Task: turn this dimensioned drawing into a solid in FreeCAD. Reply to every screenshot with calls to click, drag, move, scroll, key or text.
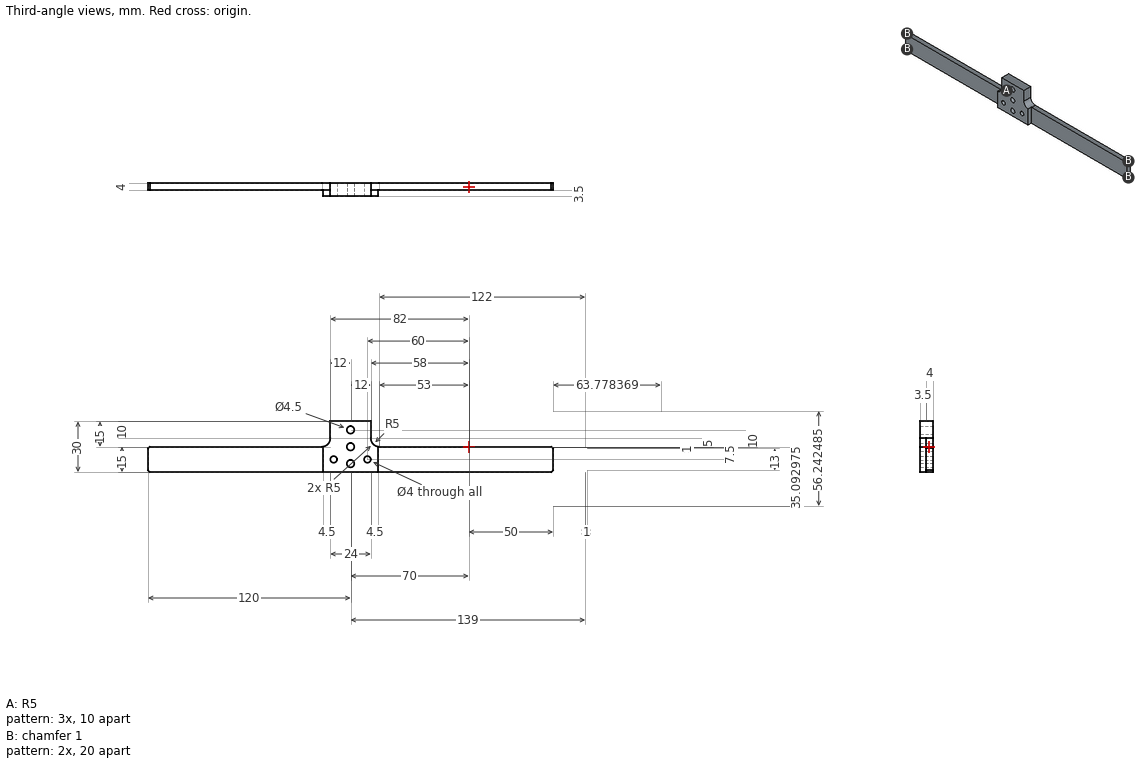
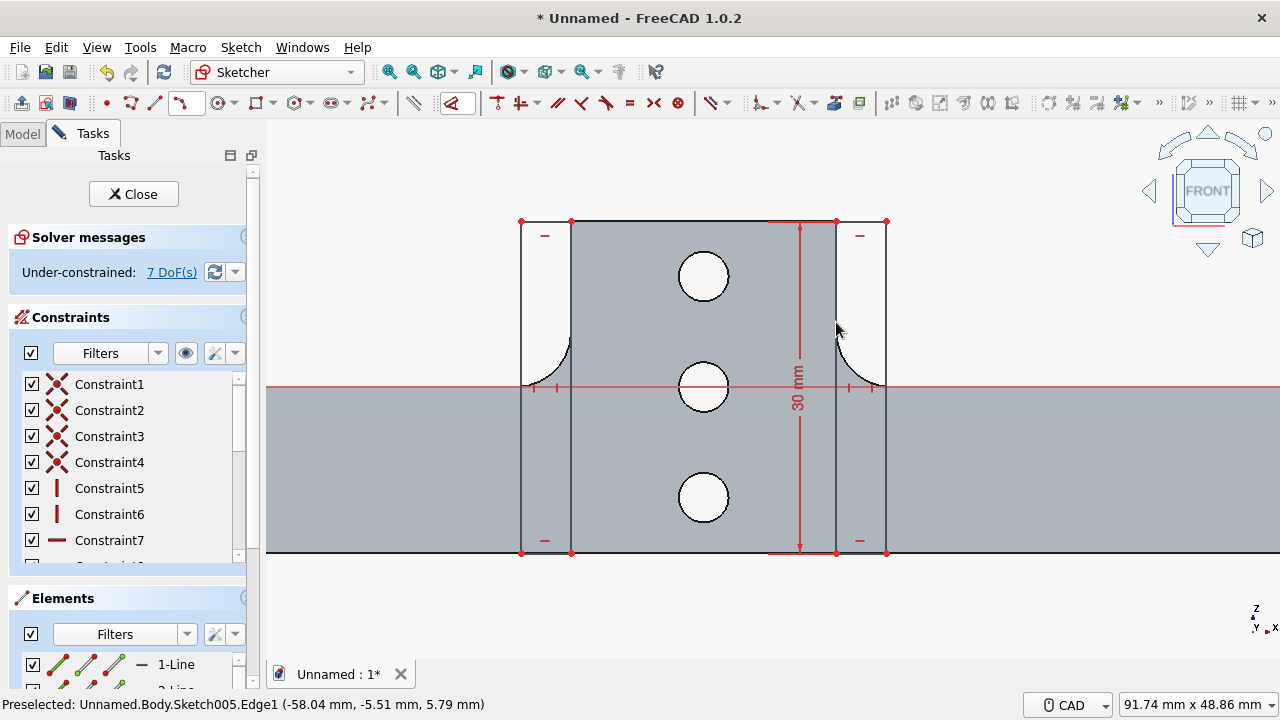
click(521, 322)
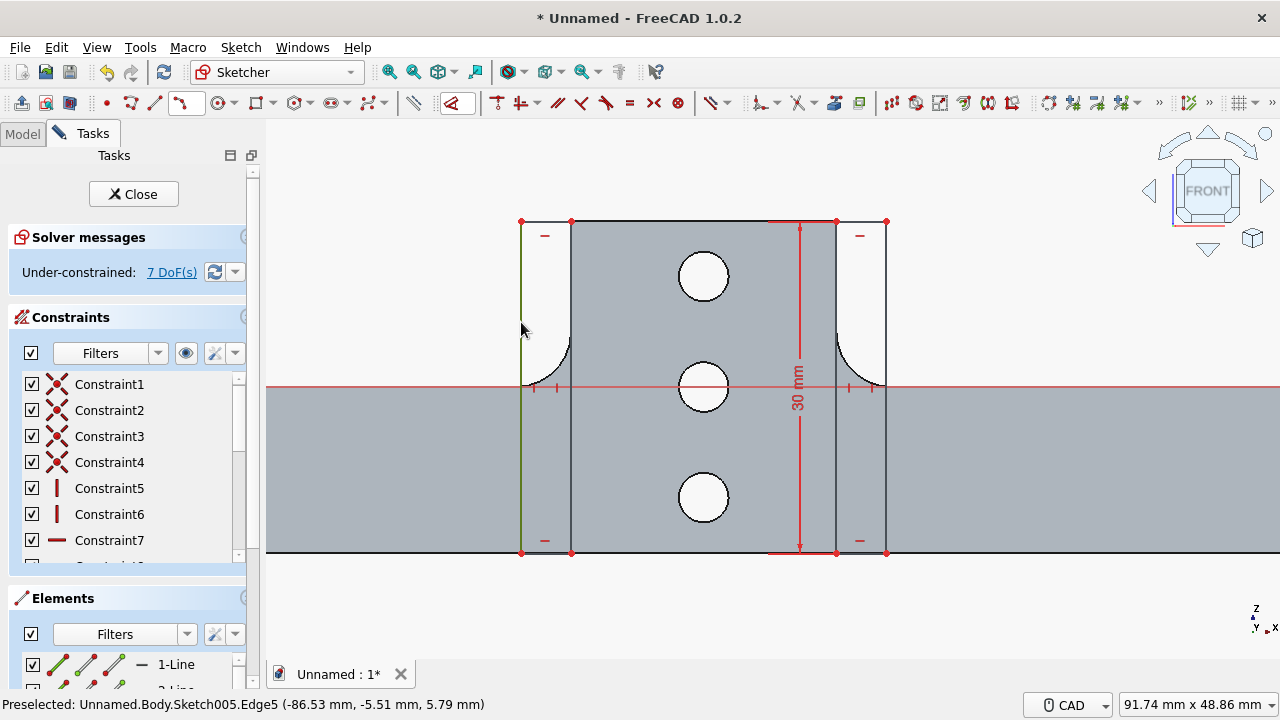
click(470, 104)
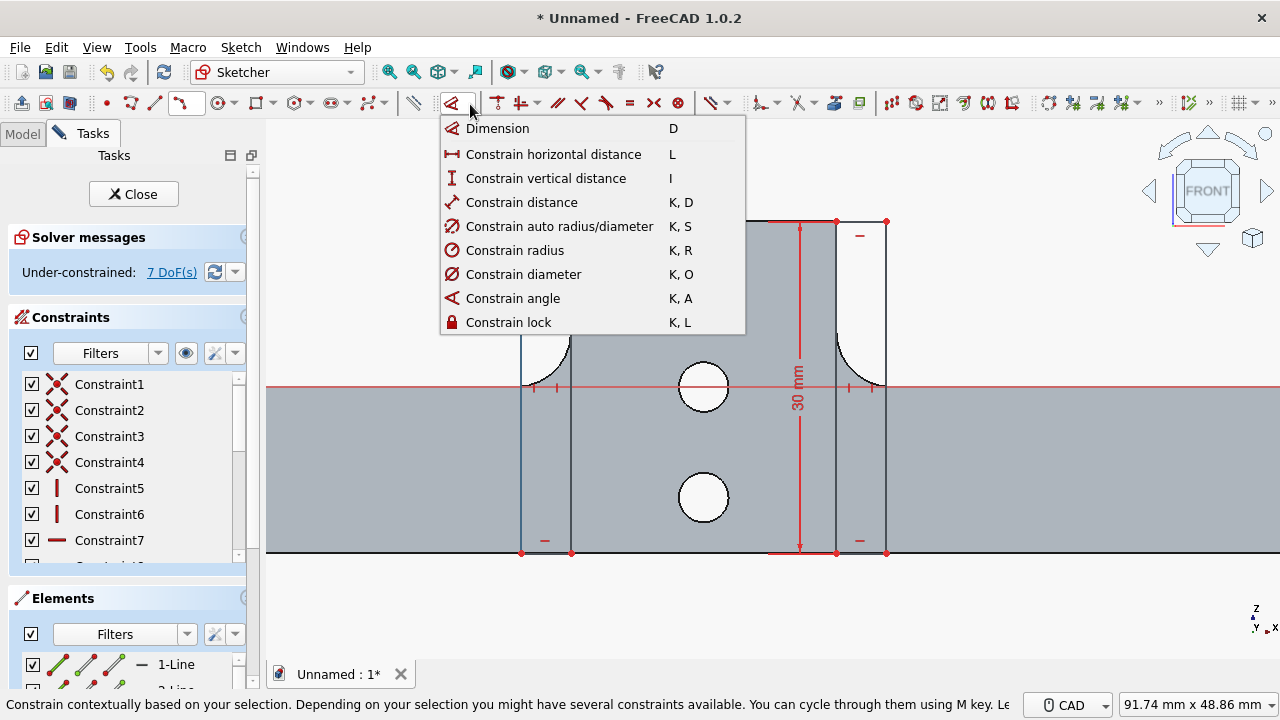
click(593, 178)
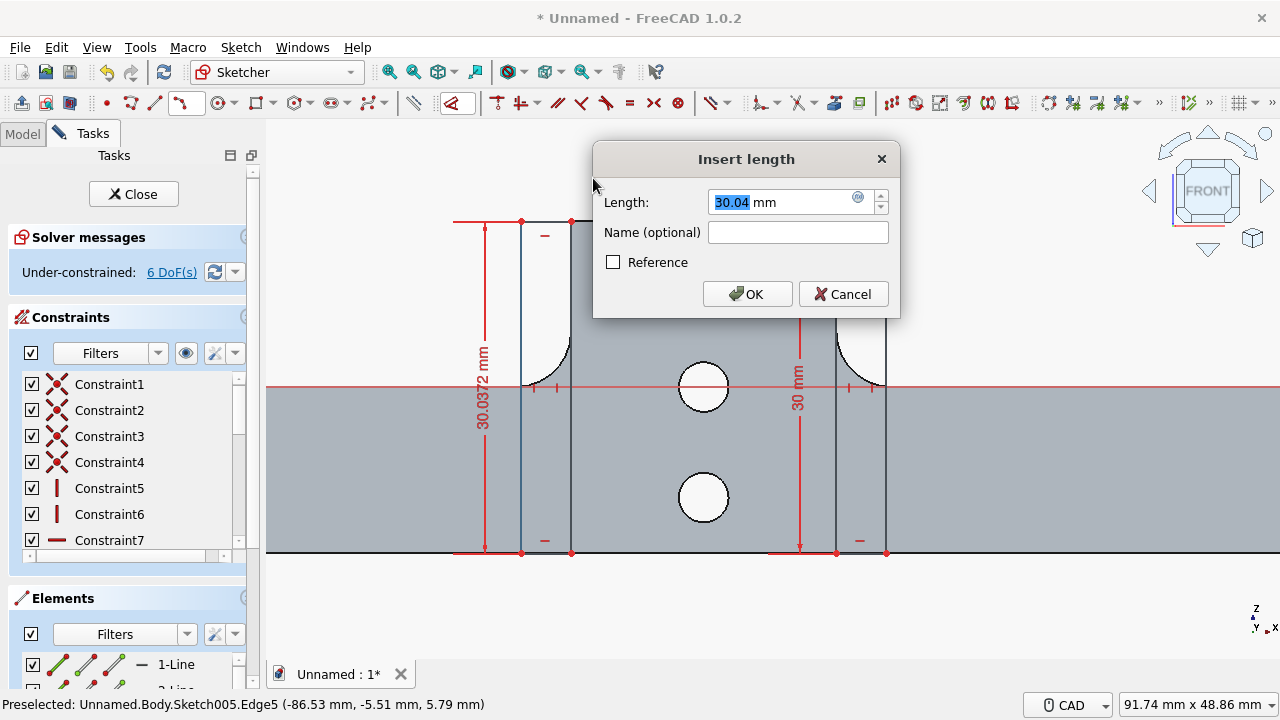
text(30)
key(Return)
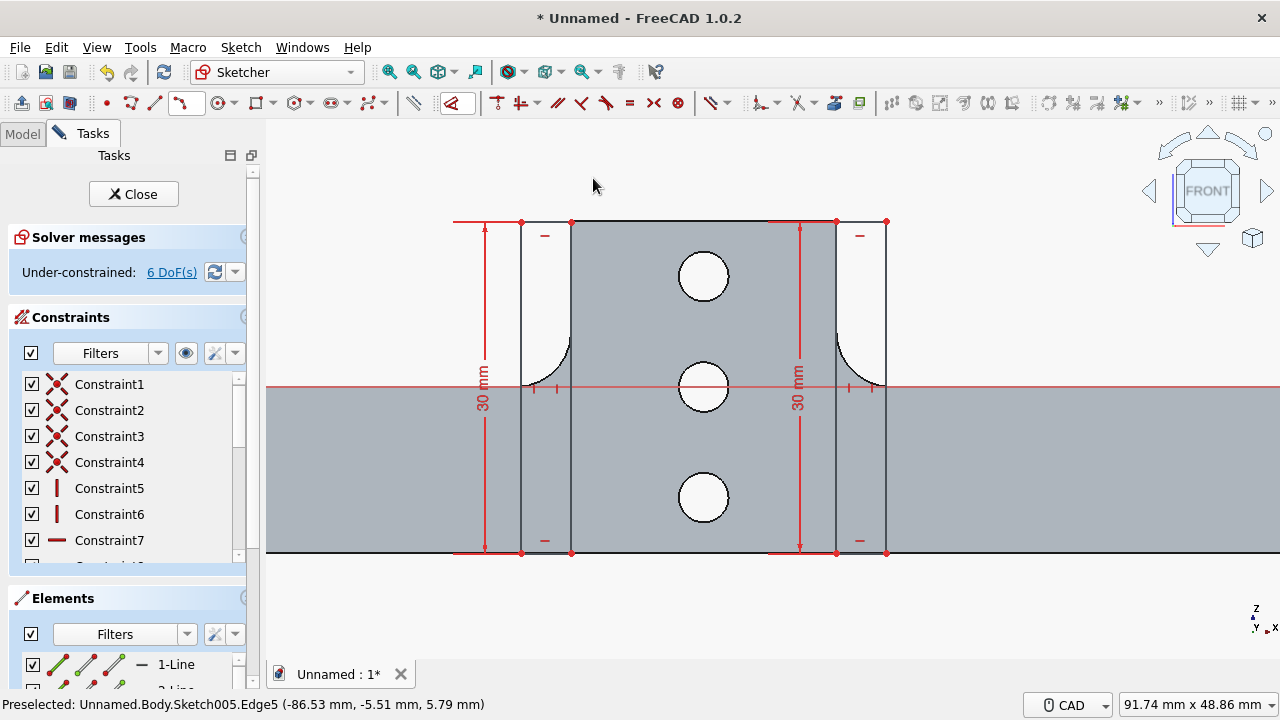
click(851, 554)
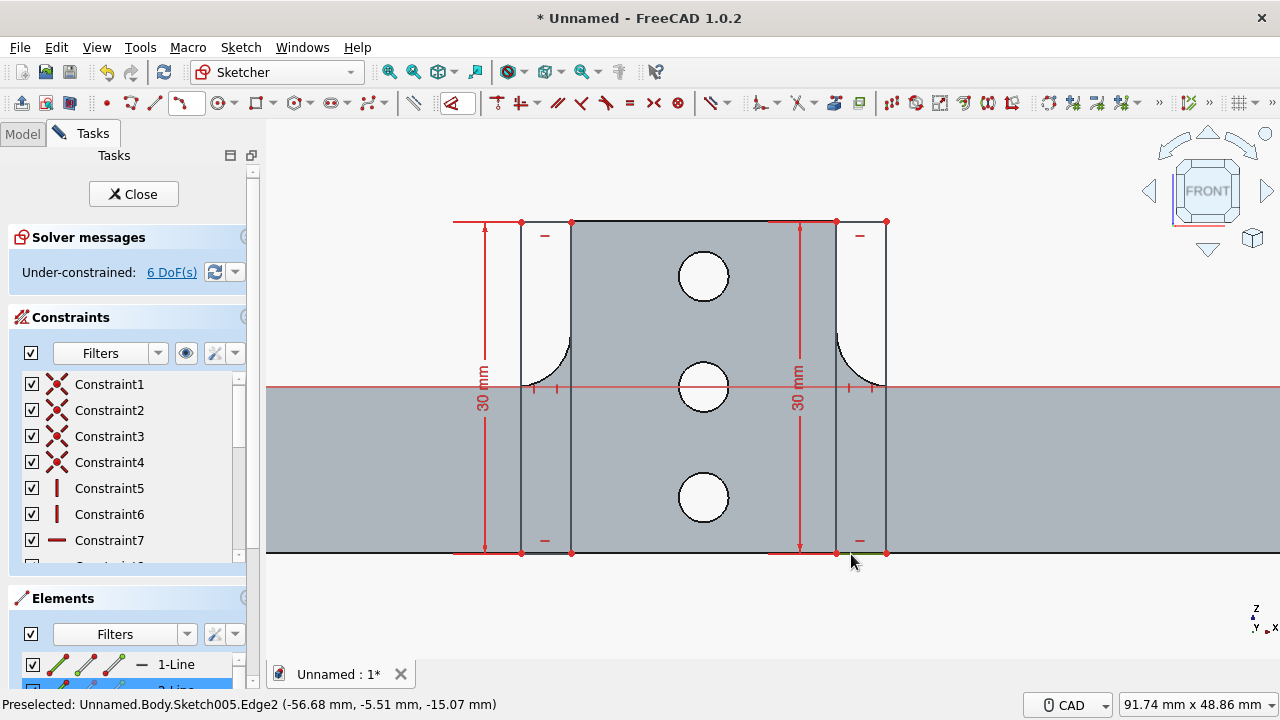
key(l)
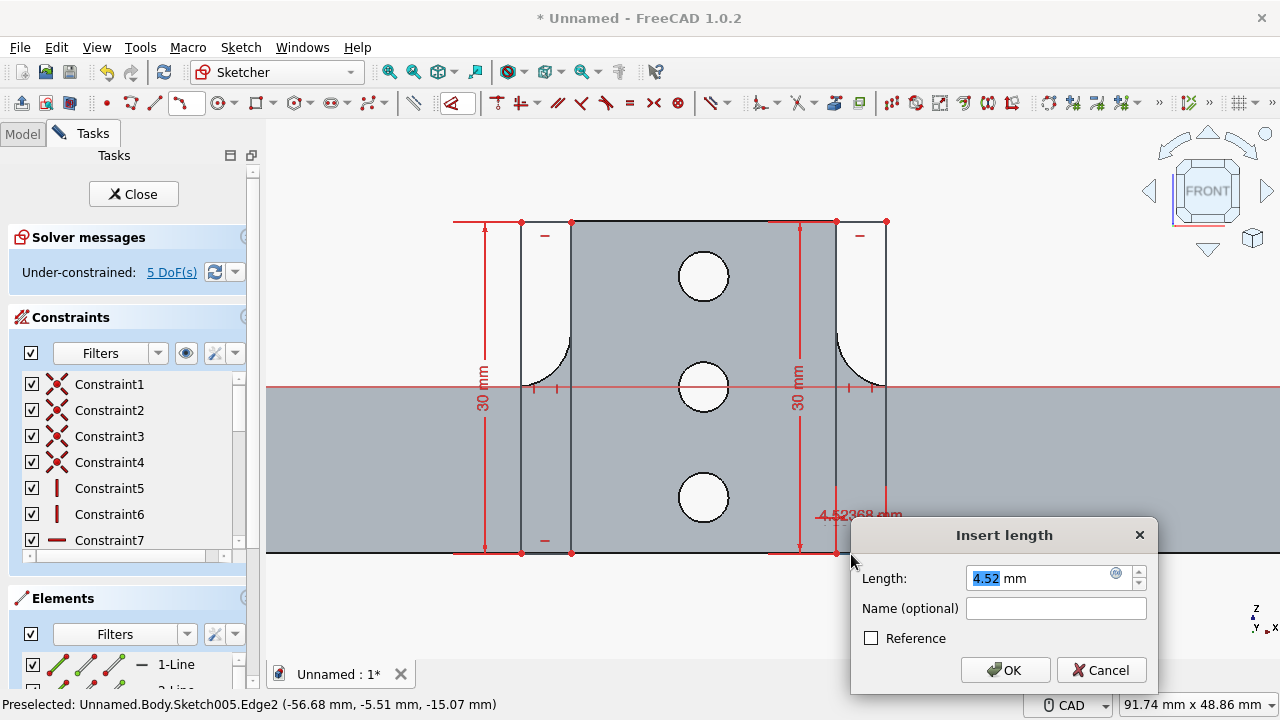
text(4.5)
key(Return)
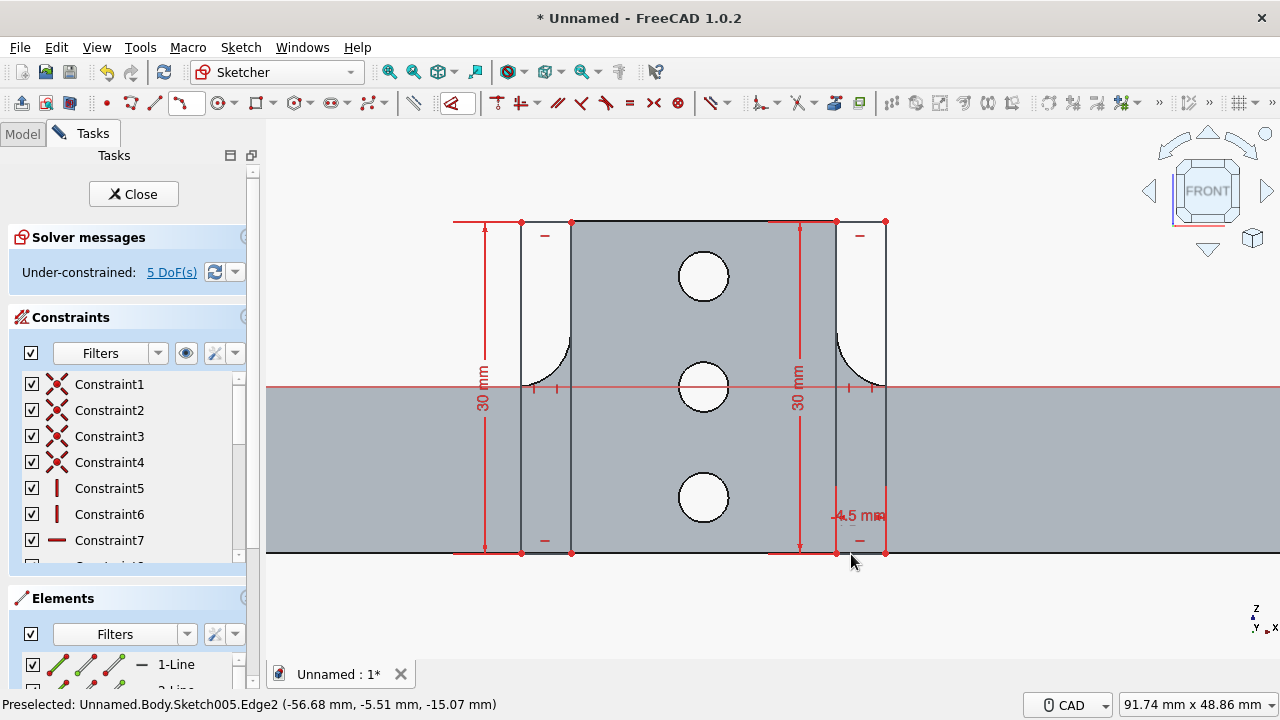
click(536, 554)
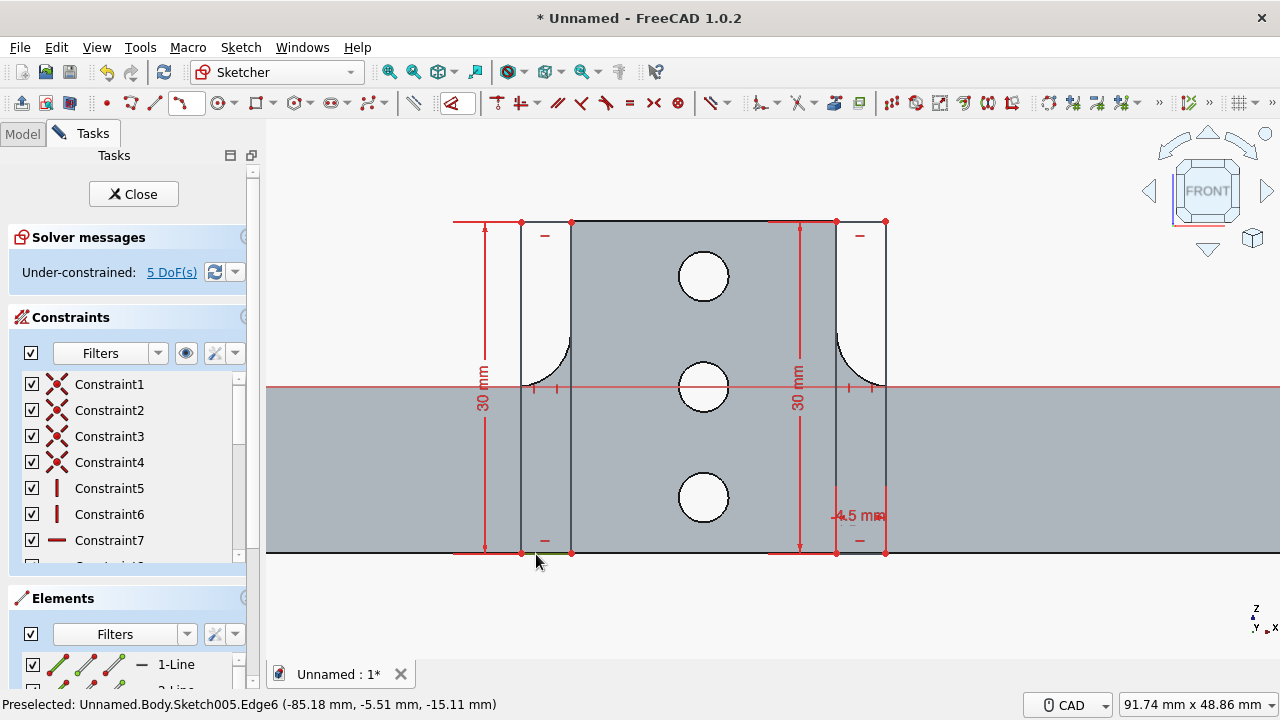
key(l)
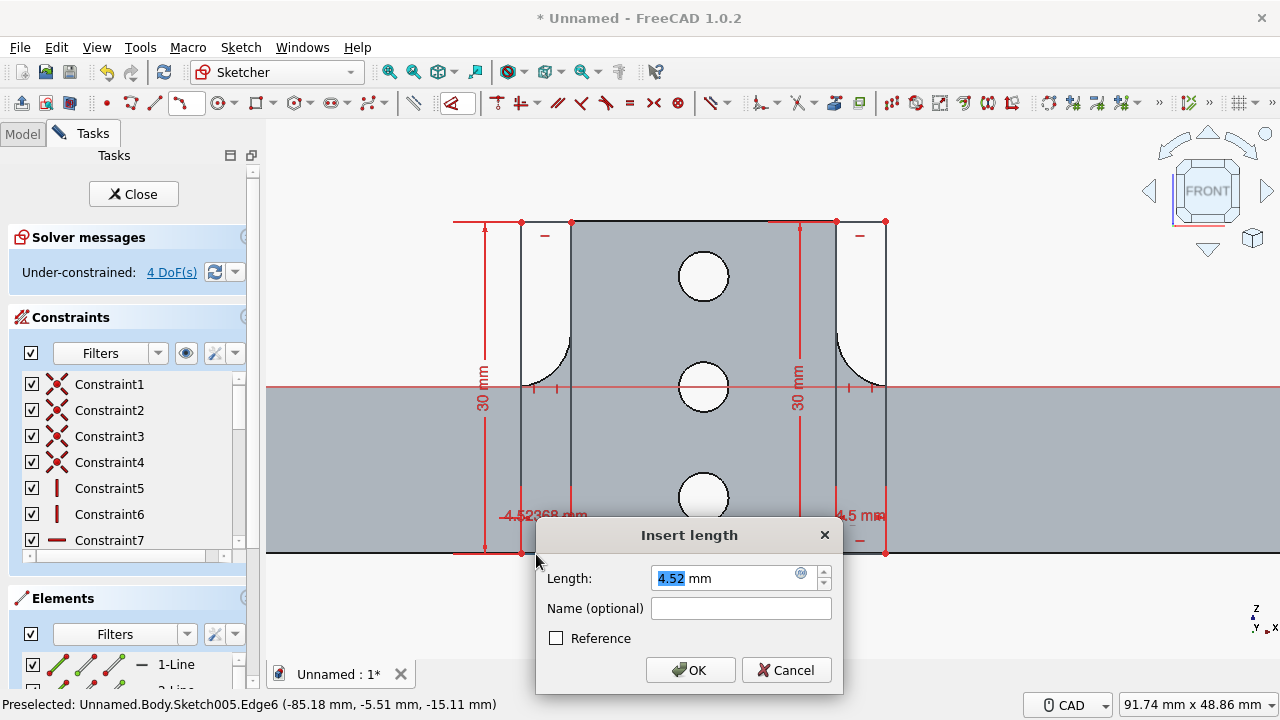
text(4.5)
key(Return)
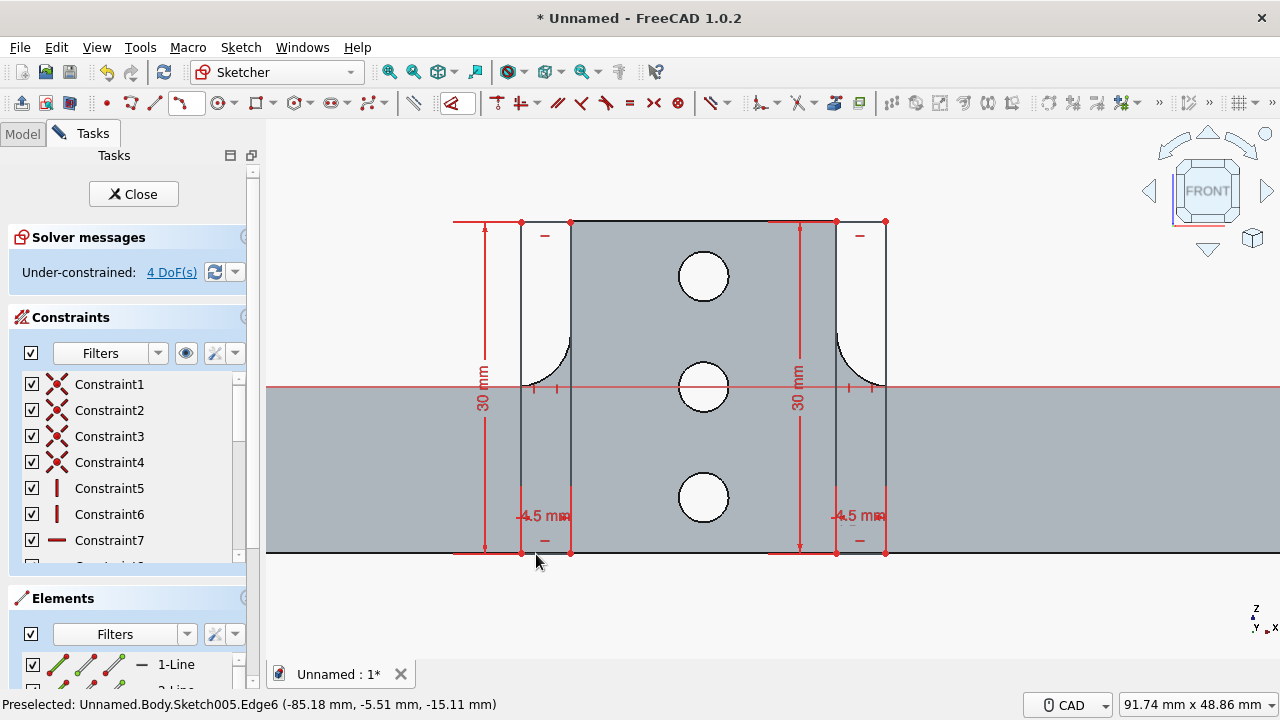
click(836, 222)